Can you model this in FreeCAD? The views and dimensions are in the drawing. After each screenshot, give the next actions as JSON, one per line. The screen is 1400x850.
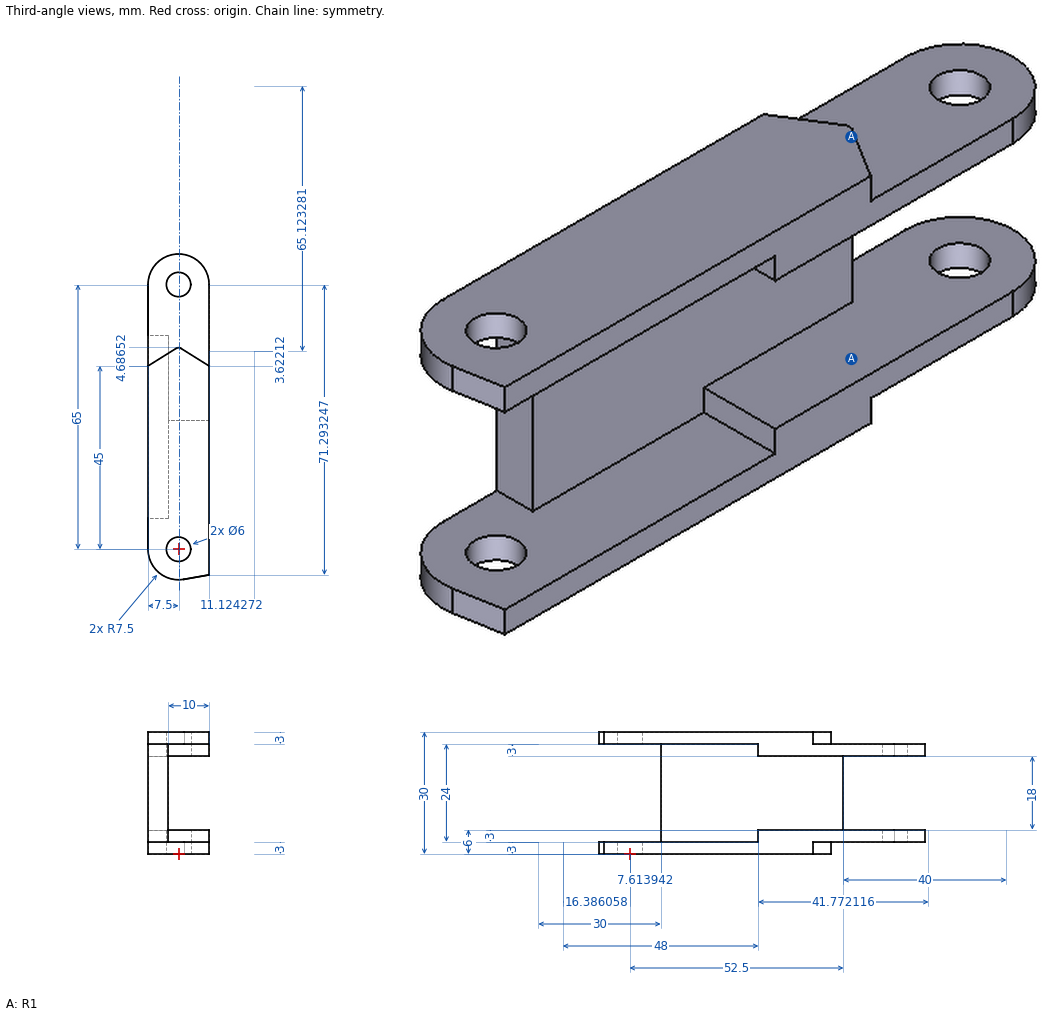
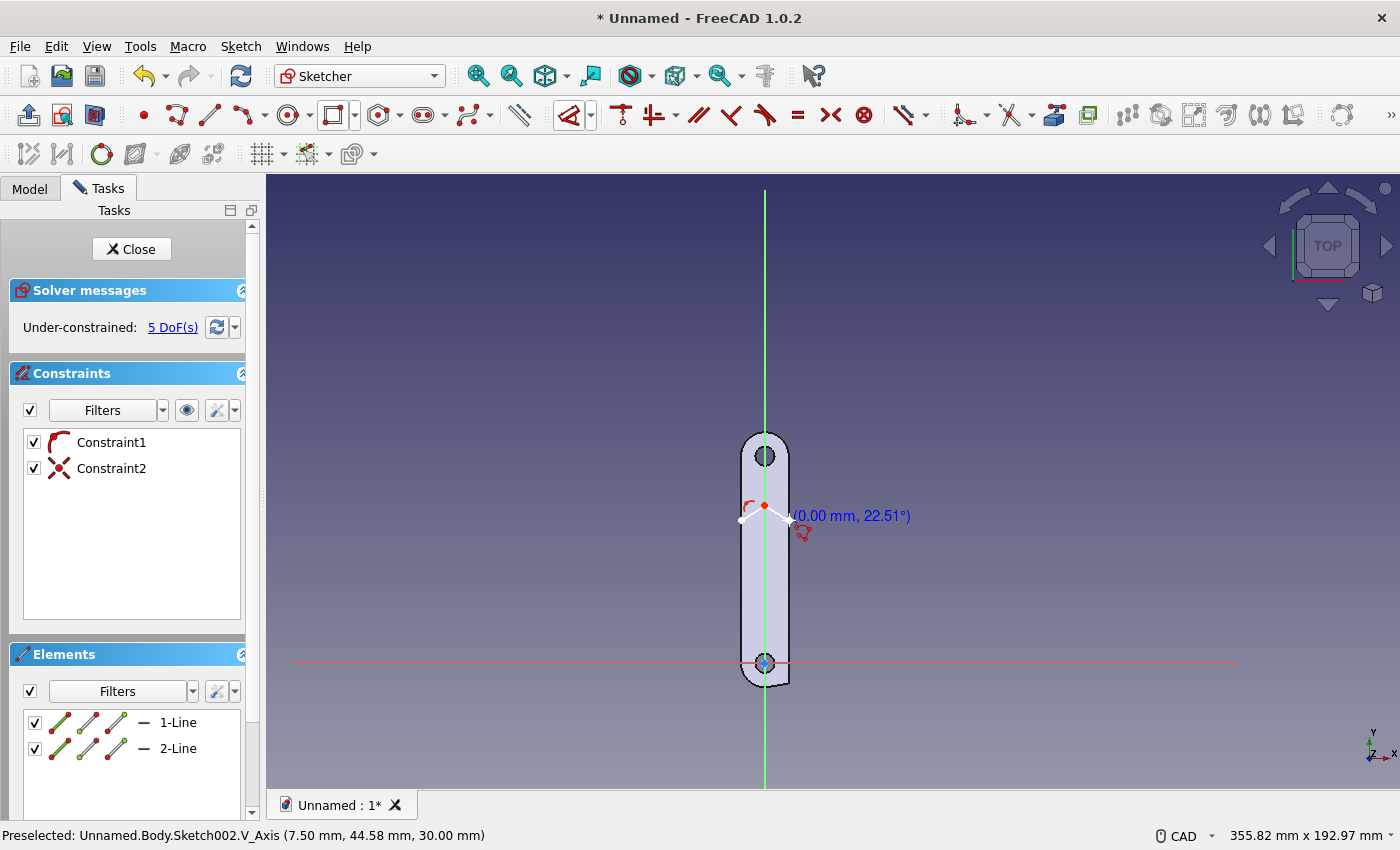
{"action": "scroll", "coordinate": [789, 508], "scroll_direction": "up", "scroll_amount": 3}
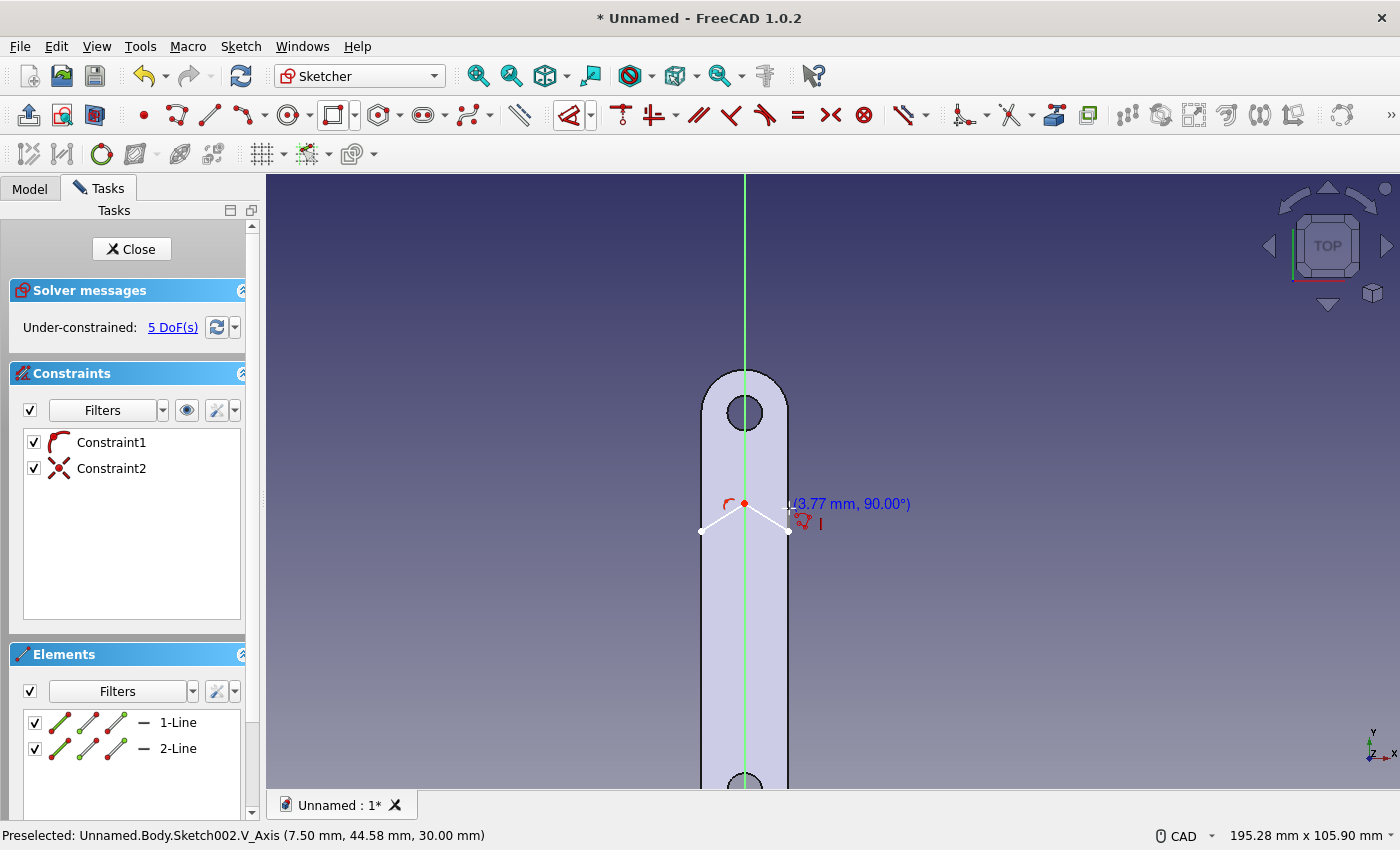
{"action": "left_click", "coordinate": [789, 508]}
{"action": "left_click", "coordinate": [853, 508]}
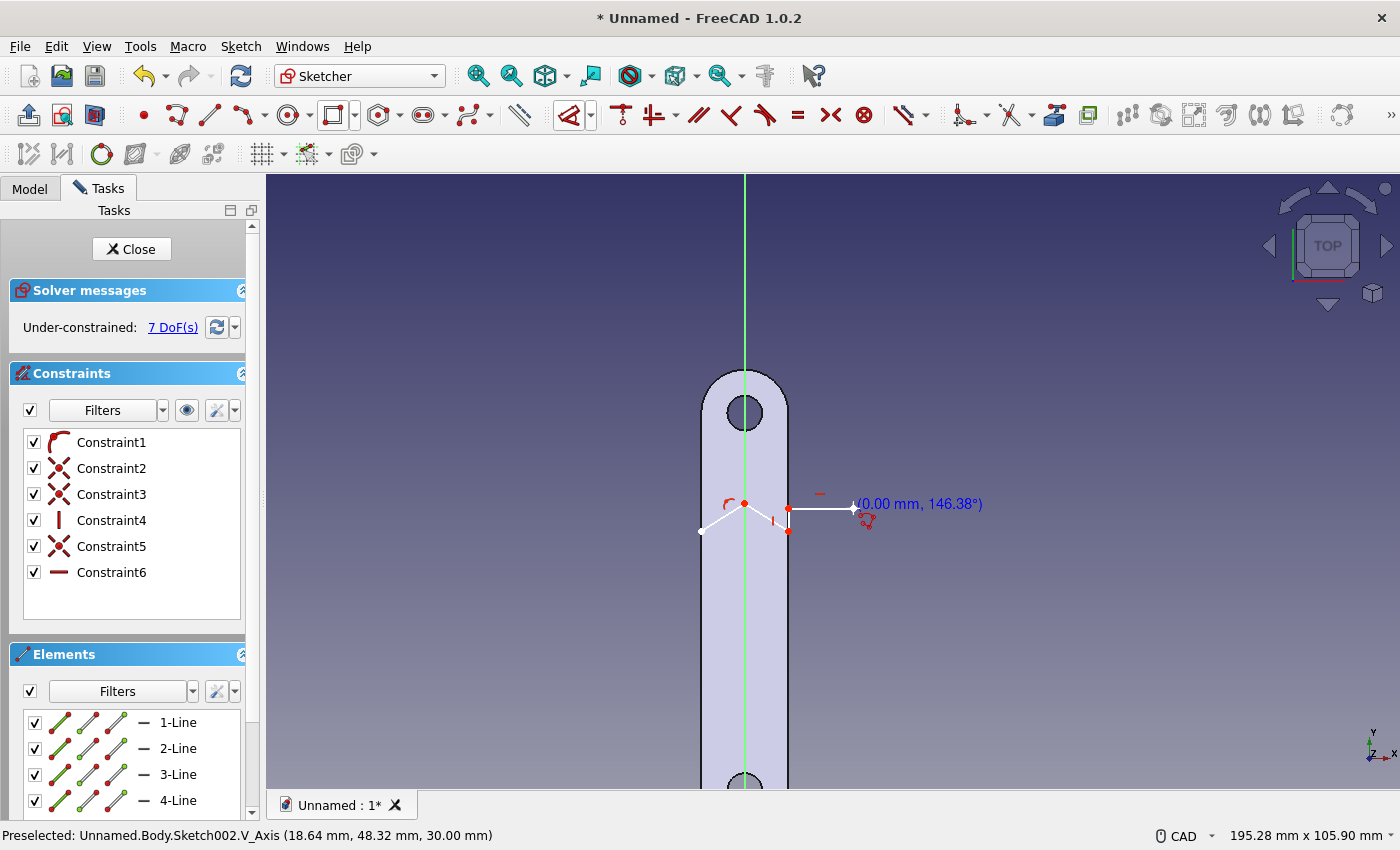
{"action": "scroll", "coordinate": [789, 507], "scroll_direction": "down", "scroll_amount": 3}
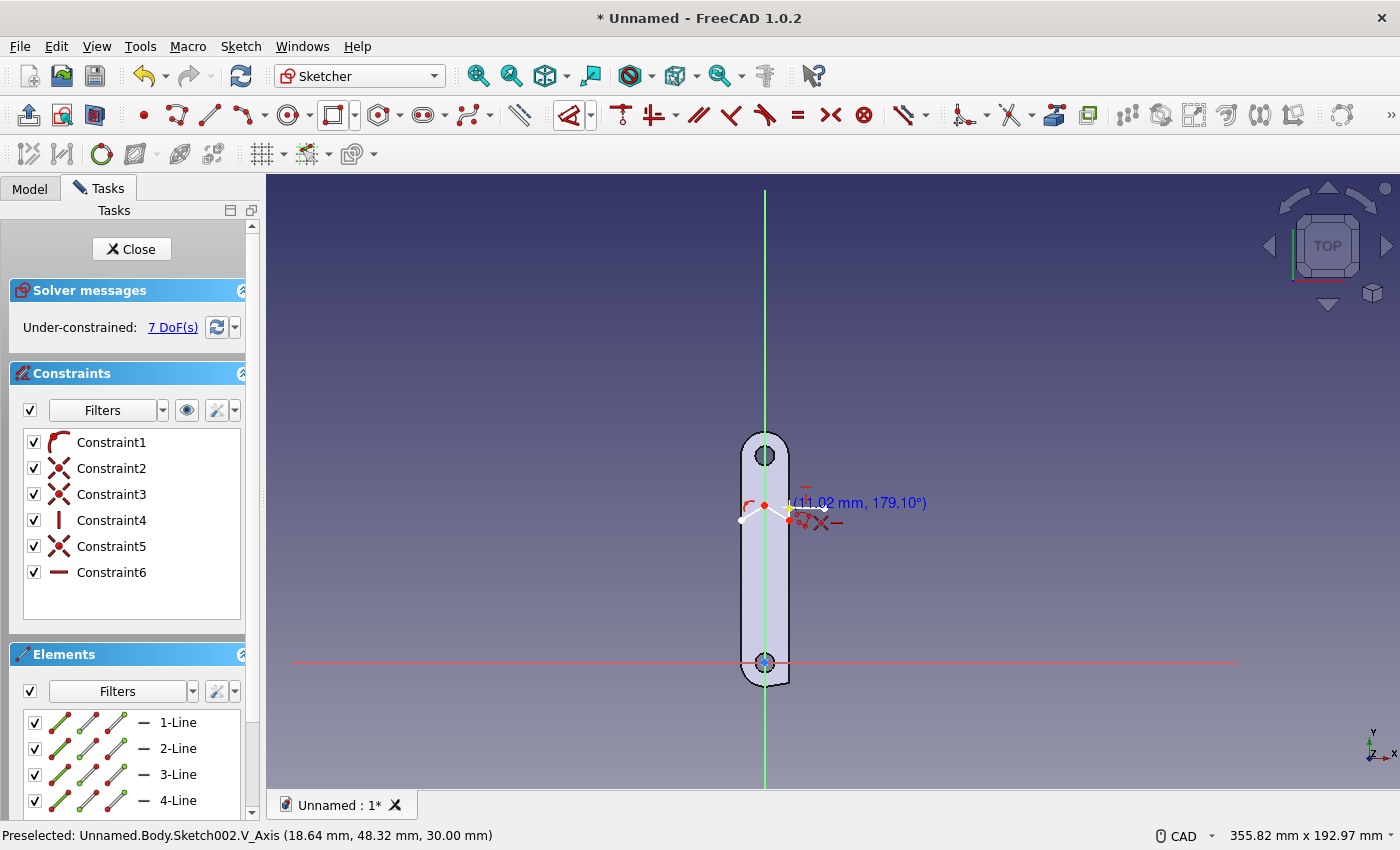
{"action": "left_click", "coordinate": [824, 300]}
{"action": "left_click", "coordinate": [706, 300]}
{"action": "left_click", "coordinate": [706, 508]}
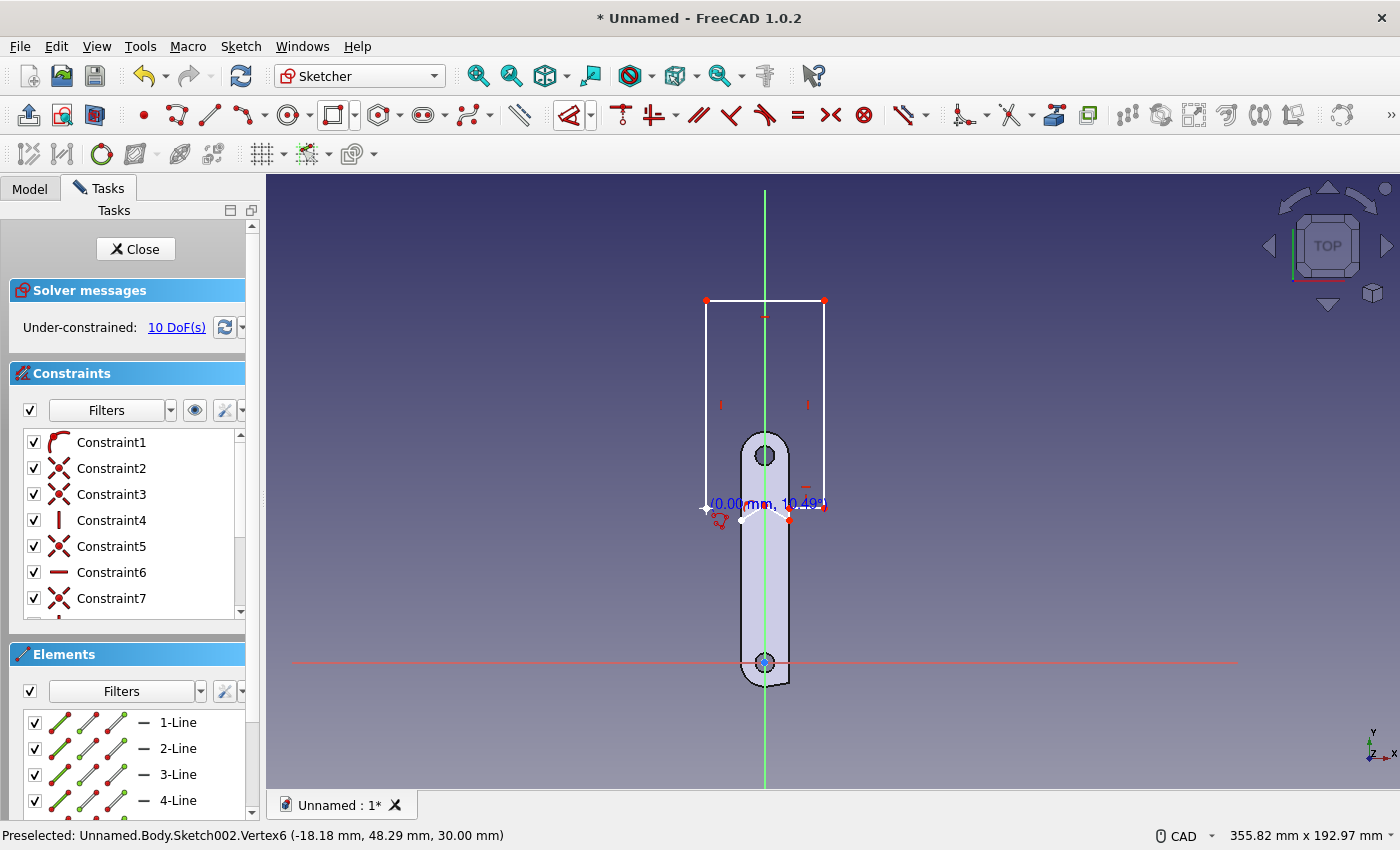
{"action": "scroll", "coordinate": [741, 508], "scroll_direction": "up", "scroll_amount": 3}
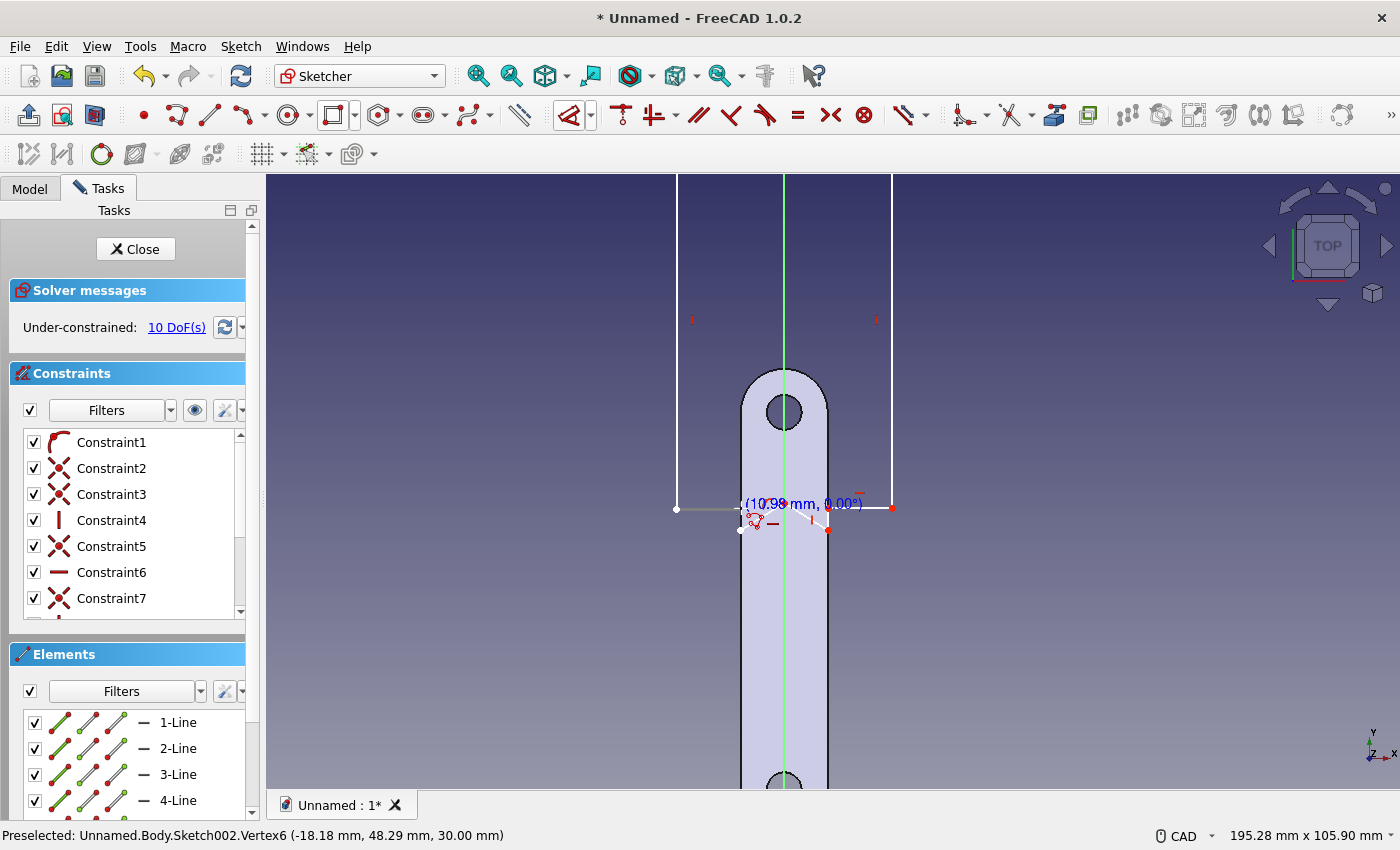
{"action": "left_click", "coordinate": [741, 508]}
{"action": "left_click", "coordinate": [741, 530]}
{"action": "key", "text": "Escape"}
{"action": "key", "text": "Escape"}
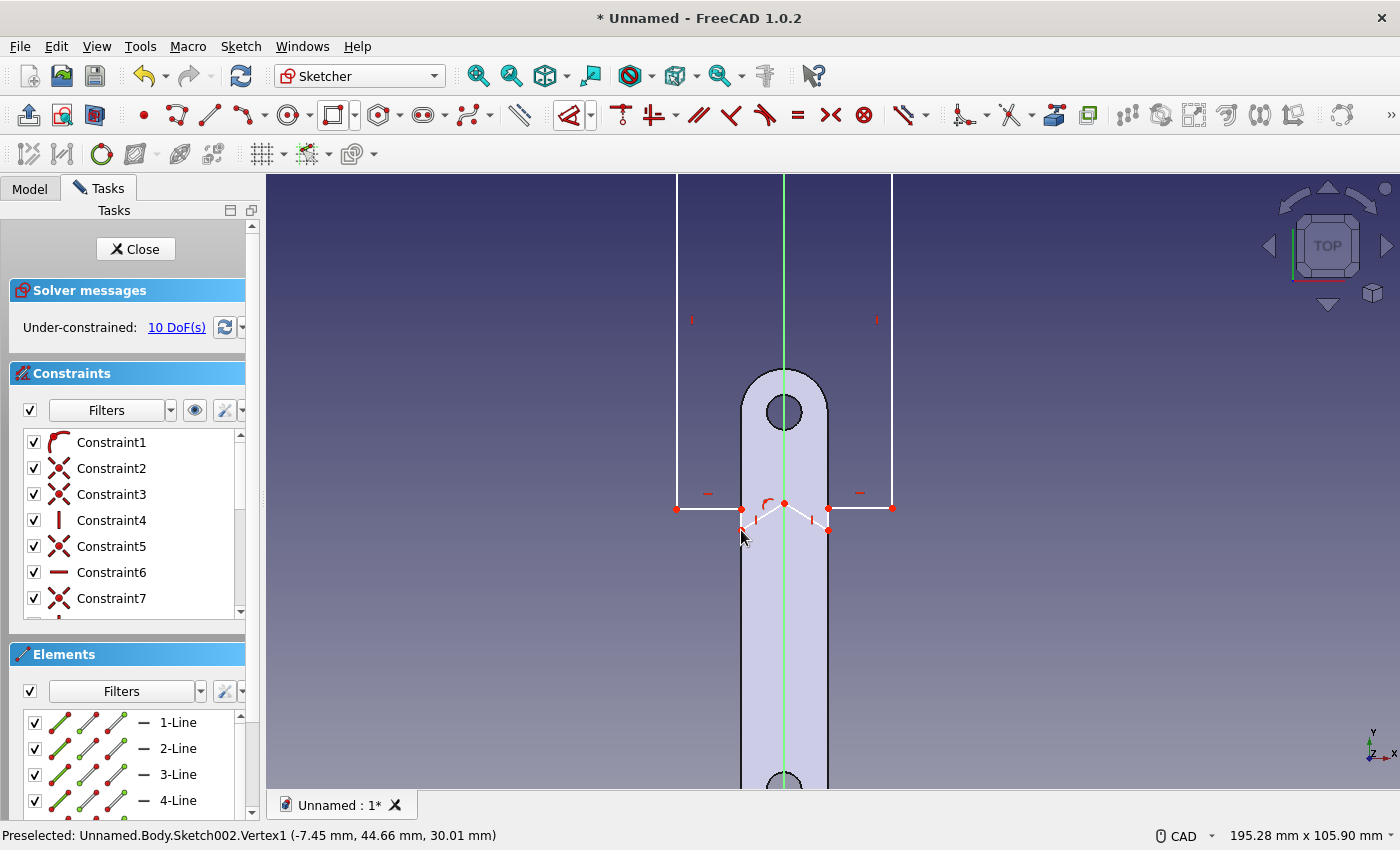
{"action": "left_click", "coordinate": [741, 530]}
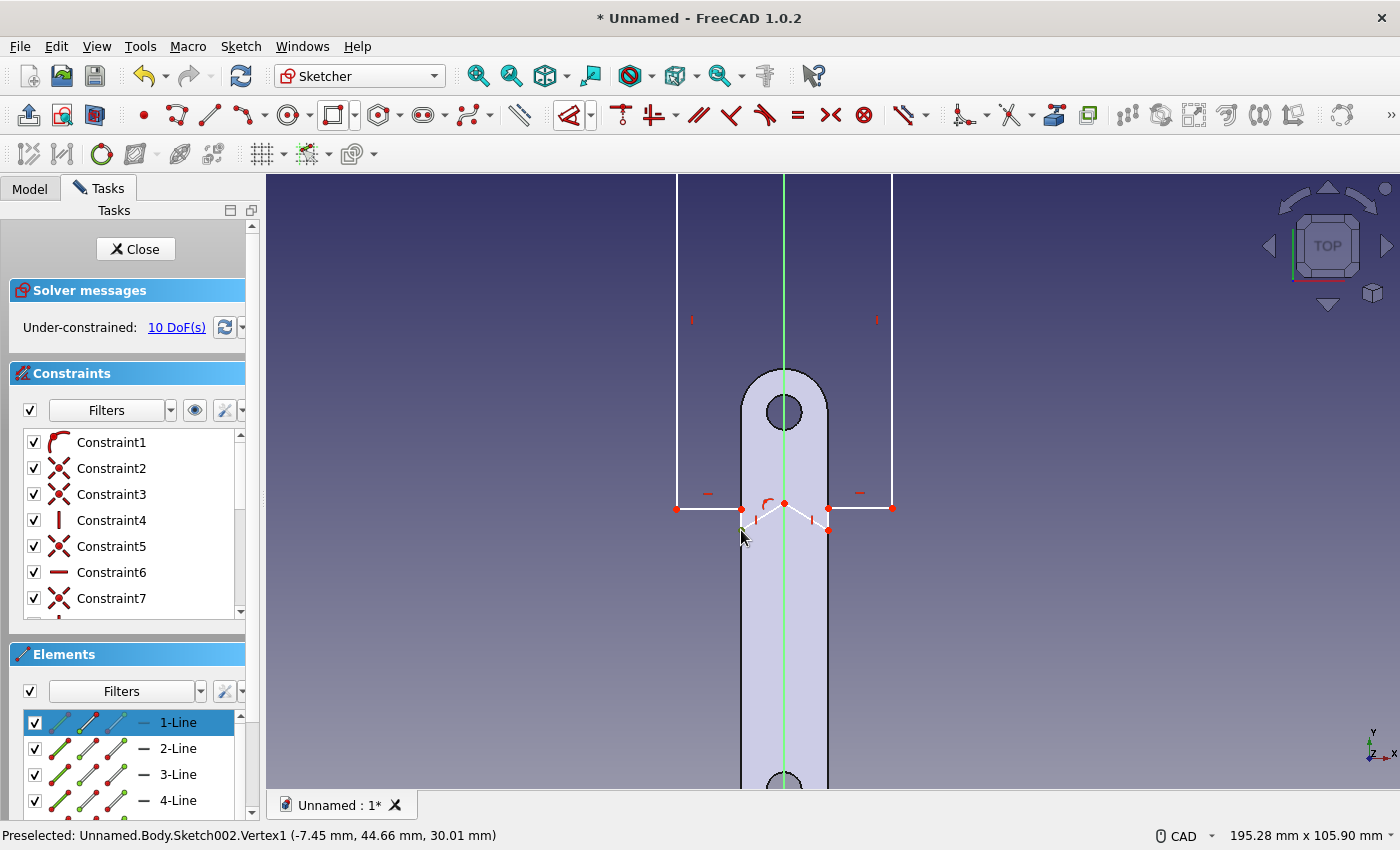
{"action": "left_click", "coordinate": [828, 530]}